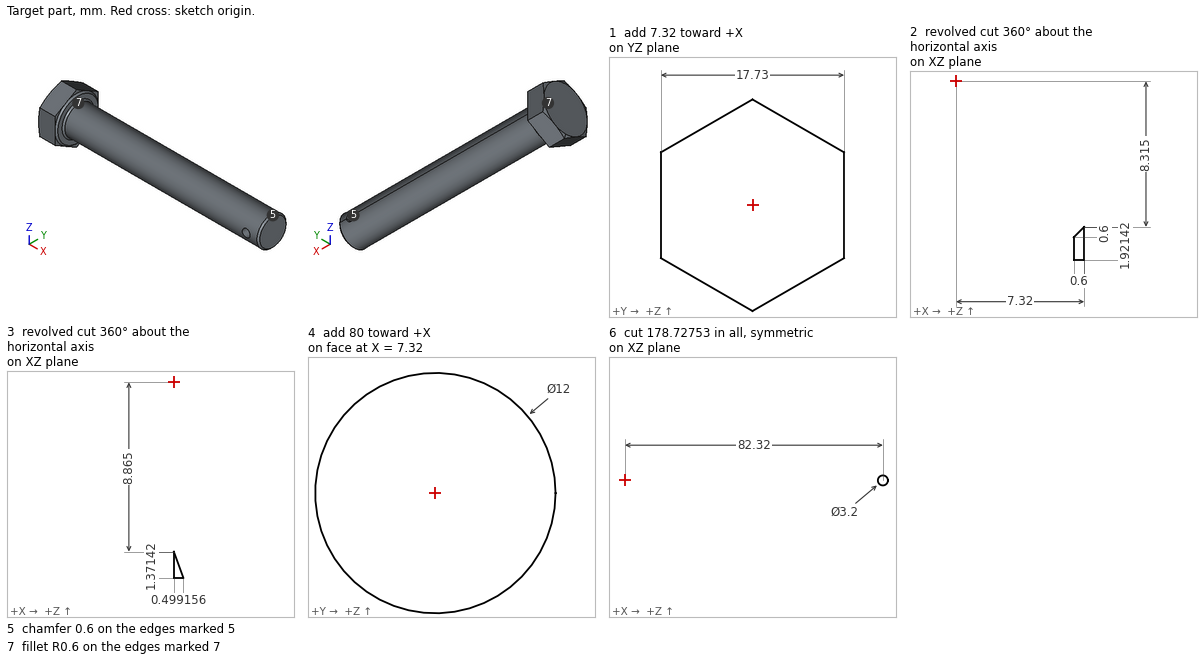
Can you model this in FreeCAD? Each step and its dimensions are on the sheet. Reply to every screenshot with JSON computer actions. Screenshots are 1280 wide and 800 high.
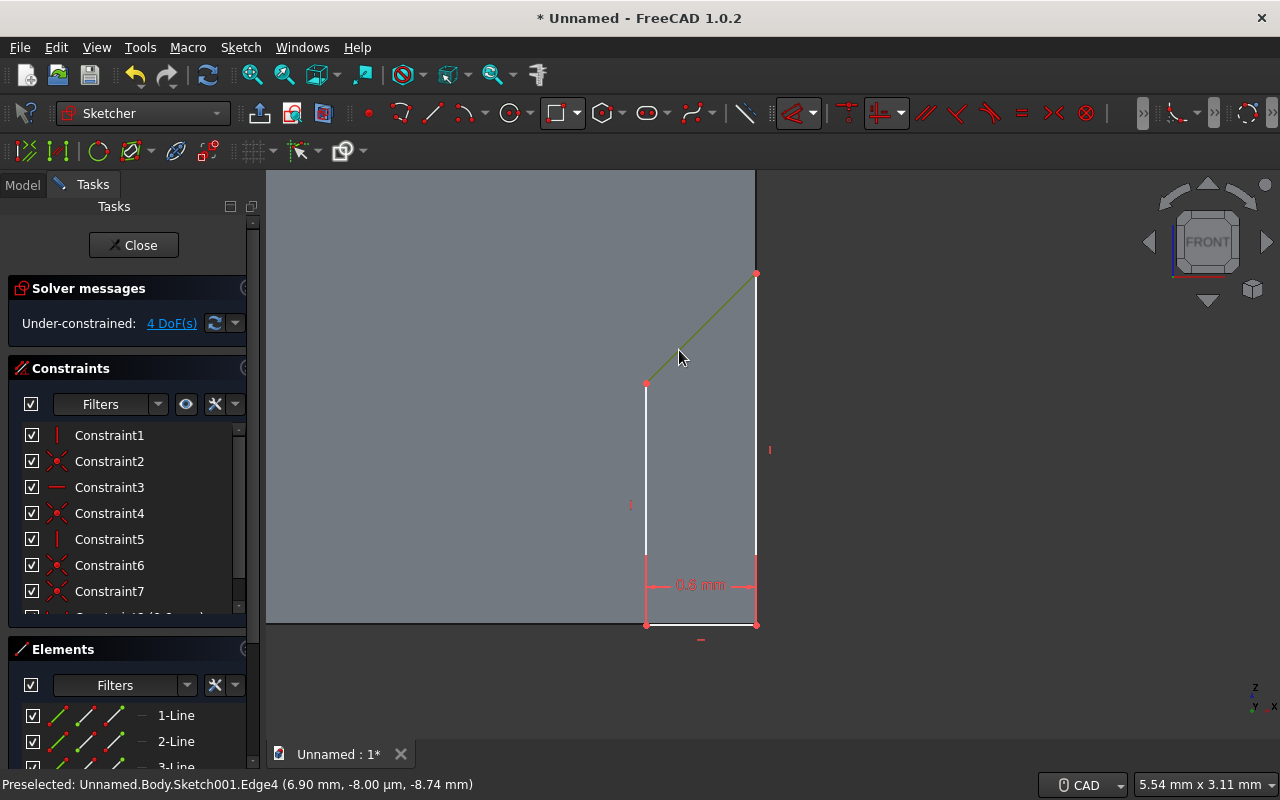
{"action": "left_click", "coordinate": [816, 114]}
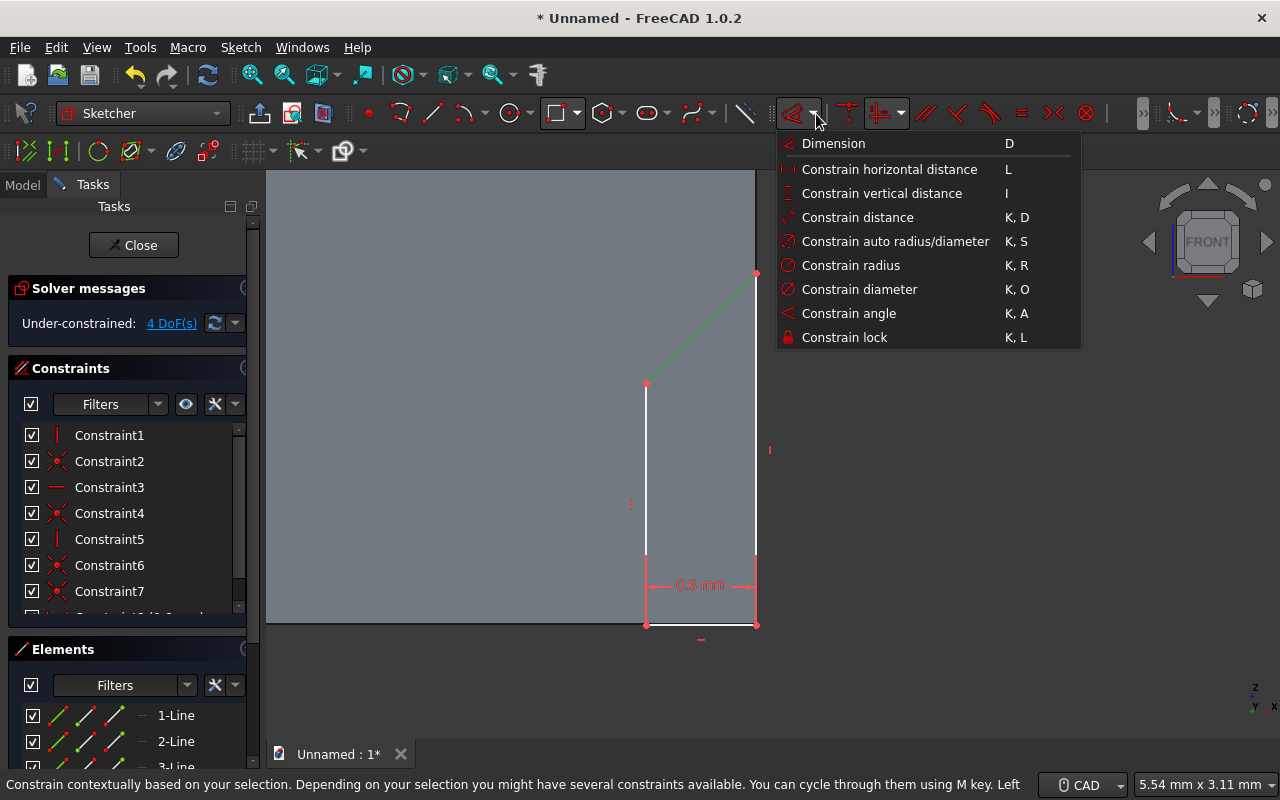
{"action": "left_click", "coordinate": [929, 193]}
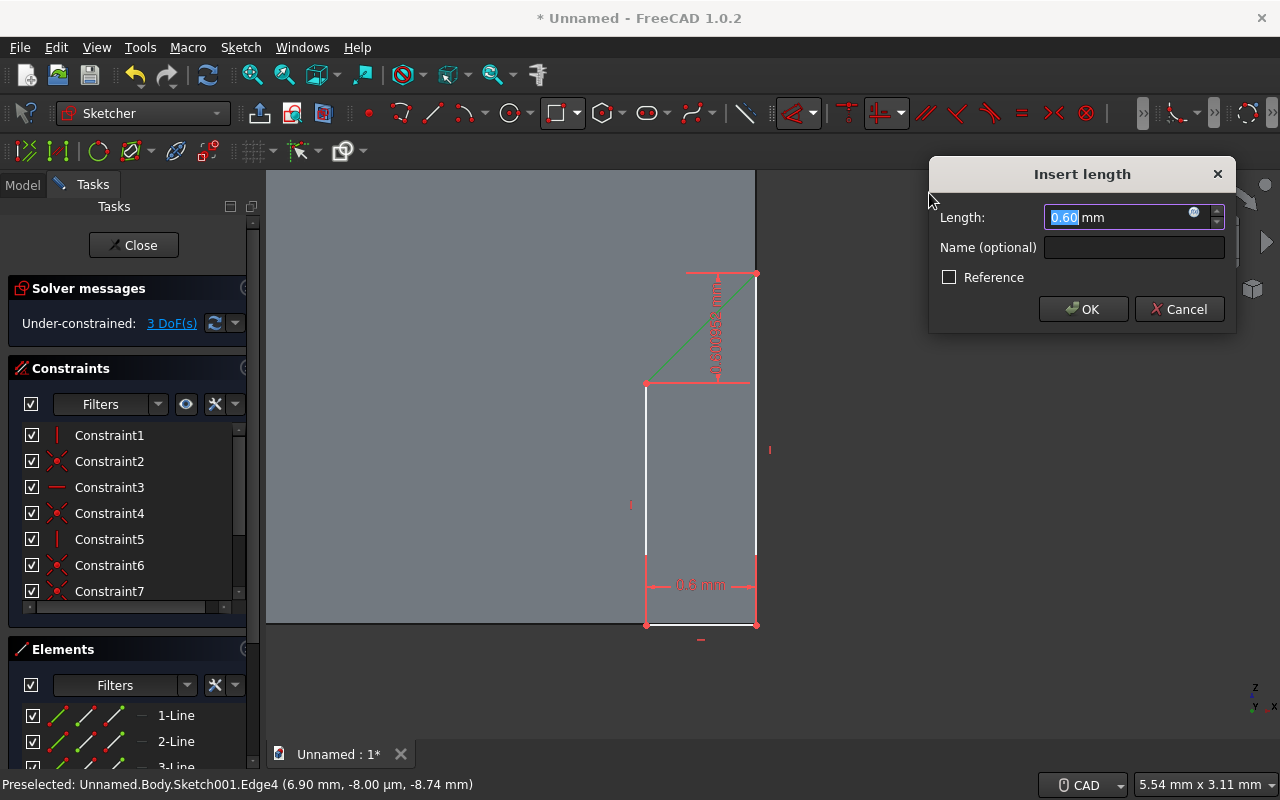
{"action": "type", "text": "0.6"}
{"action": "key", "text": "Return"}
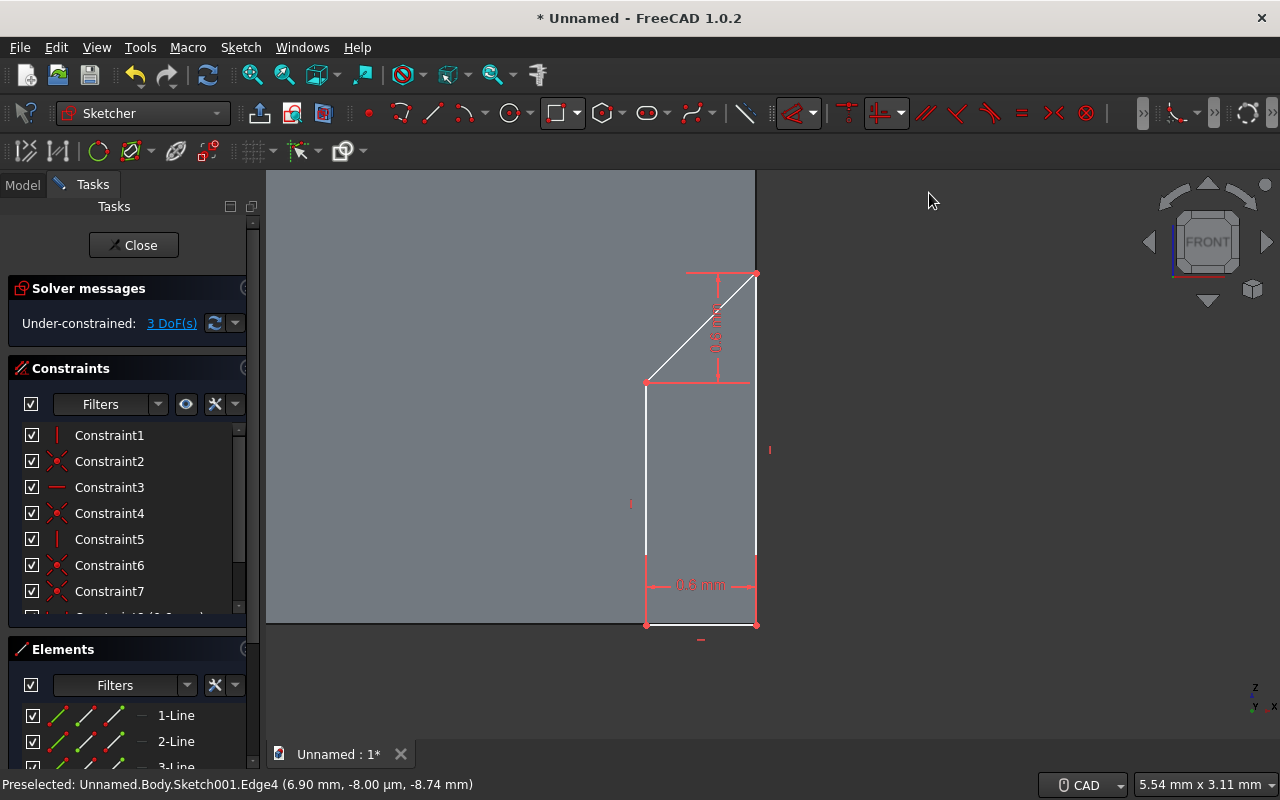
{"action": "left_click", "coordinate": [756, 273]}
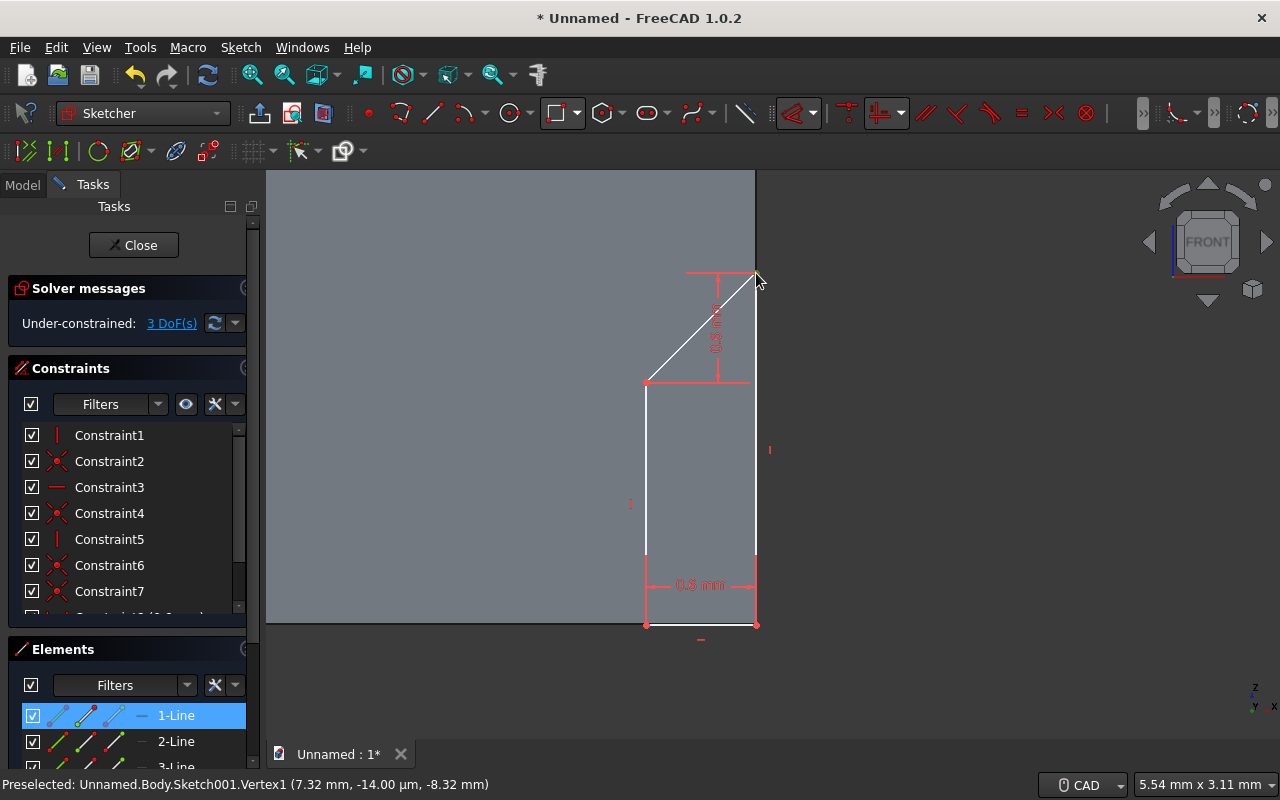
{"action": "left_click", "coordinate": [816, 114]}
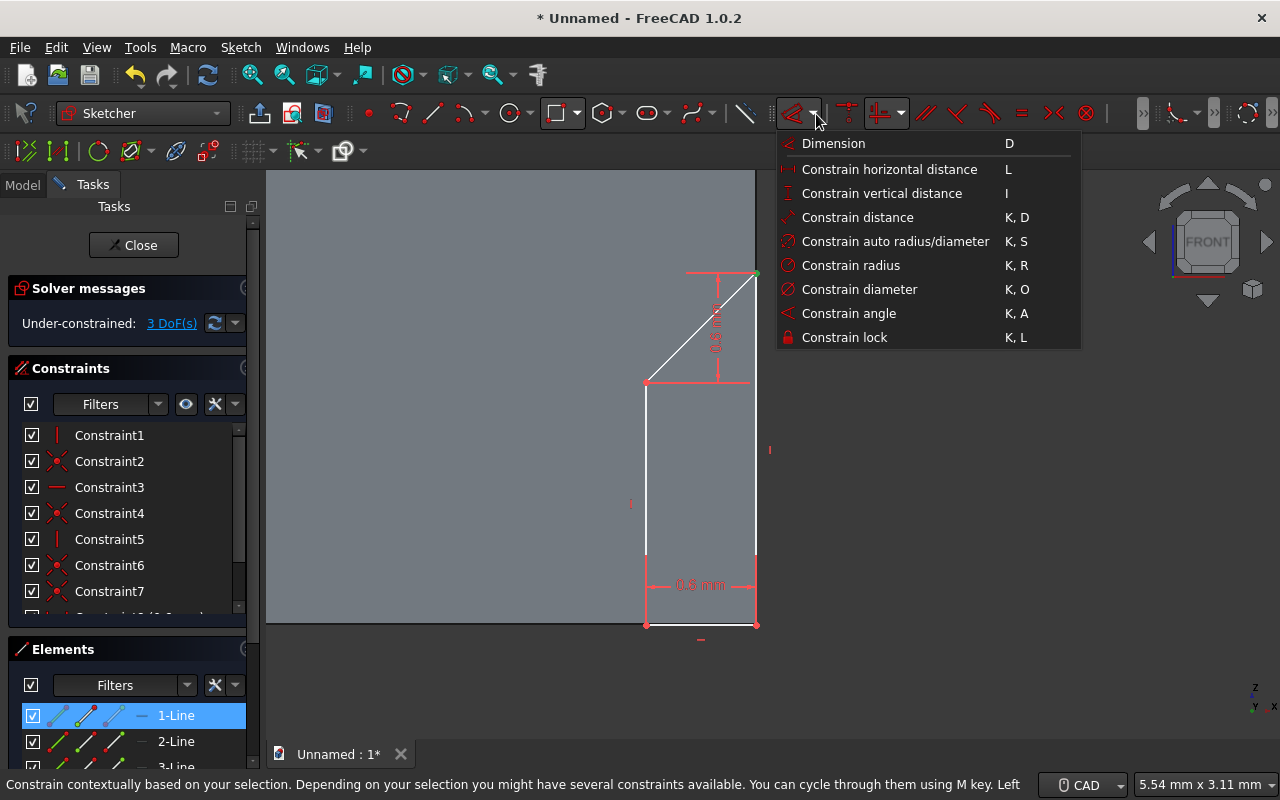
{"action": "left_click", "coordinate": [929, 169]}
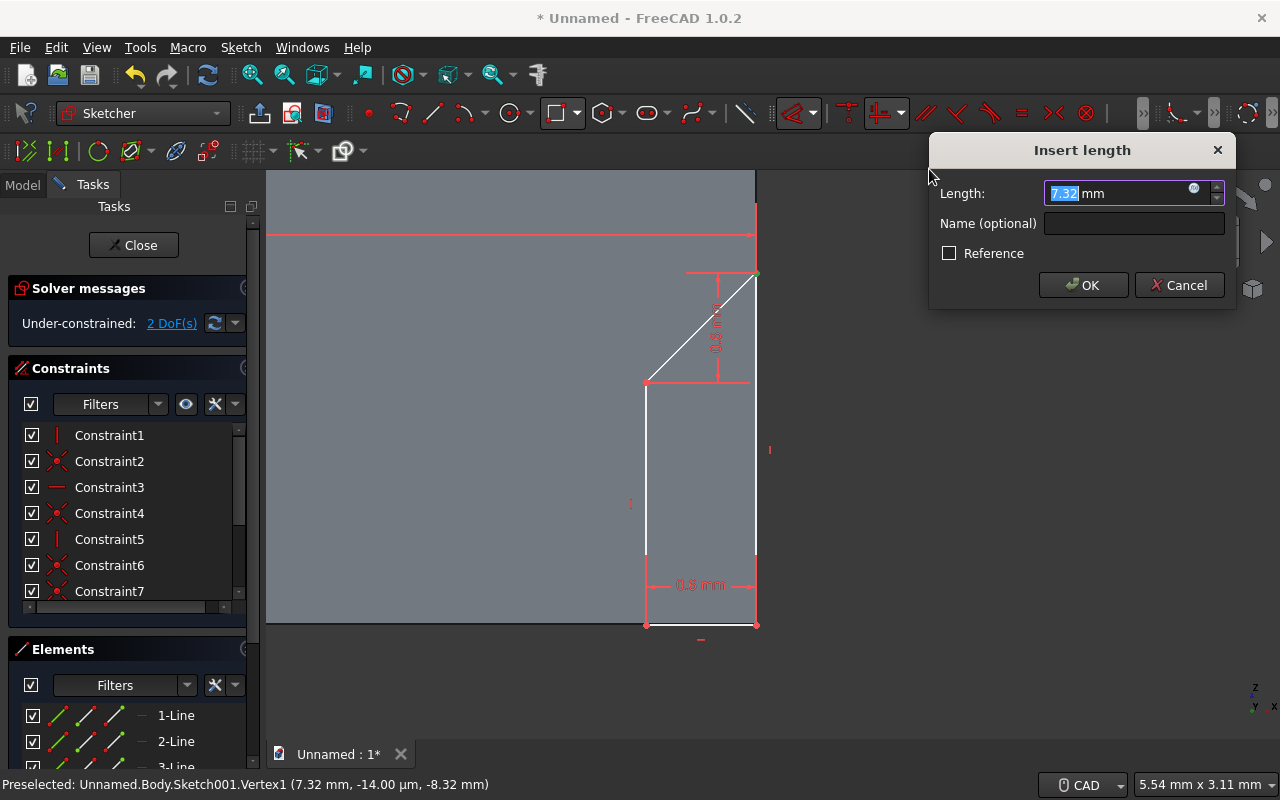
{"action": "type", "text": "7.32"}
{"action": "key", "text": "Return"}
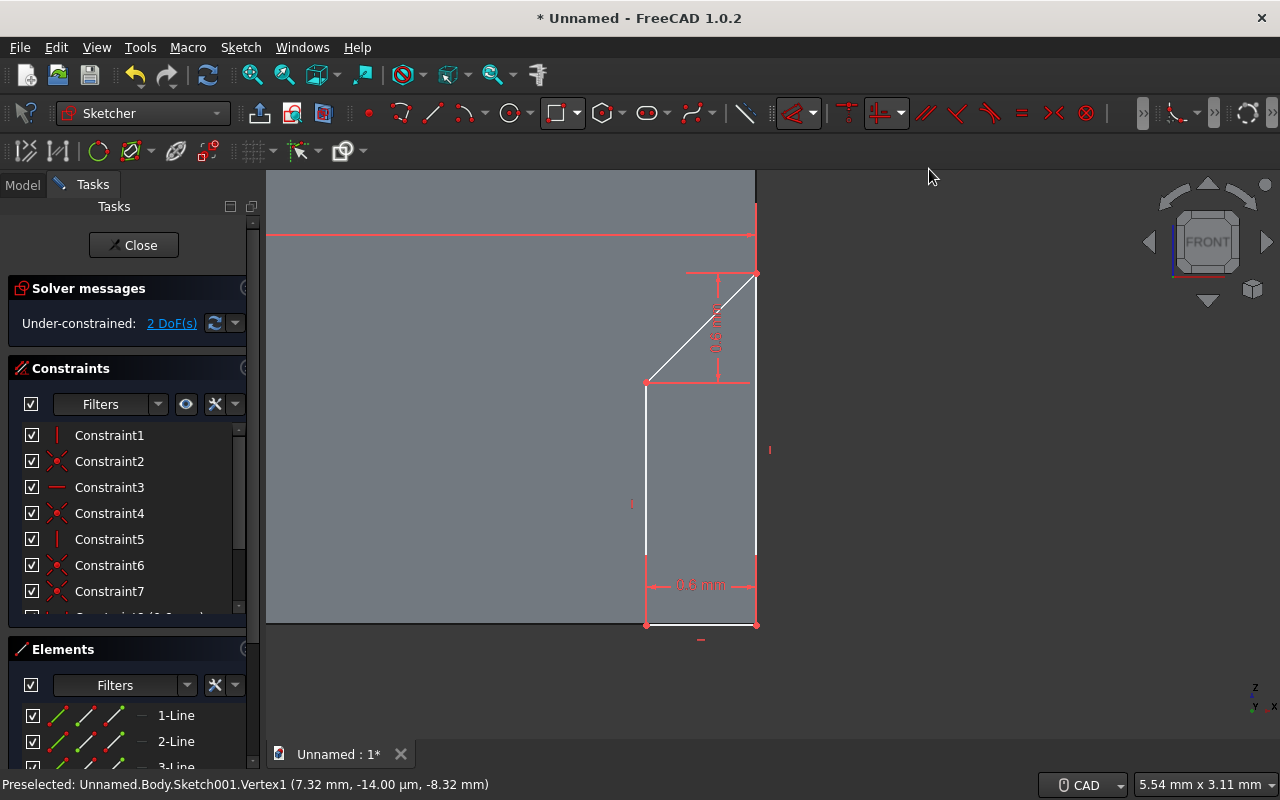
{"action": "left_click", "coordinate": [756, 273]}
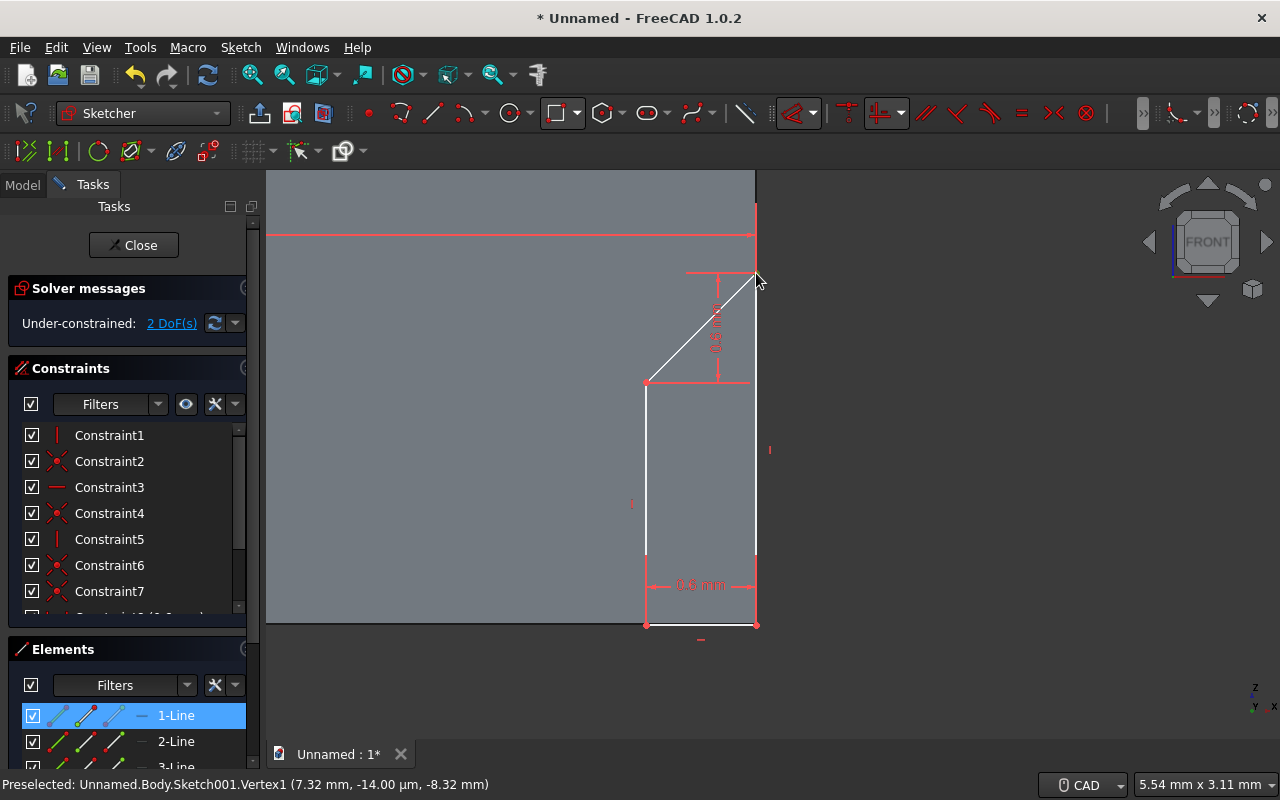
{"action": "left_click", "coordinate": [816, 114]}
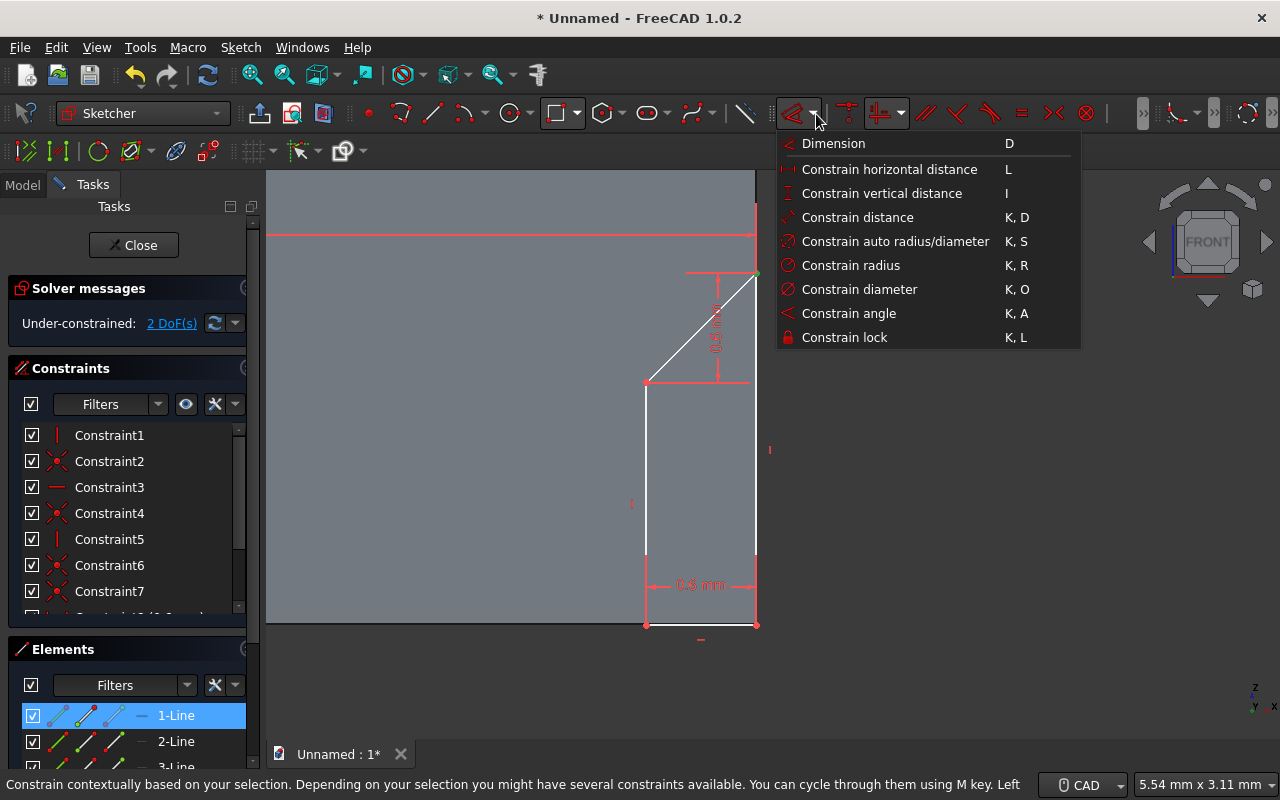
{"action": "left_click", "coordinate": [929, 193]}